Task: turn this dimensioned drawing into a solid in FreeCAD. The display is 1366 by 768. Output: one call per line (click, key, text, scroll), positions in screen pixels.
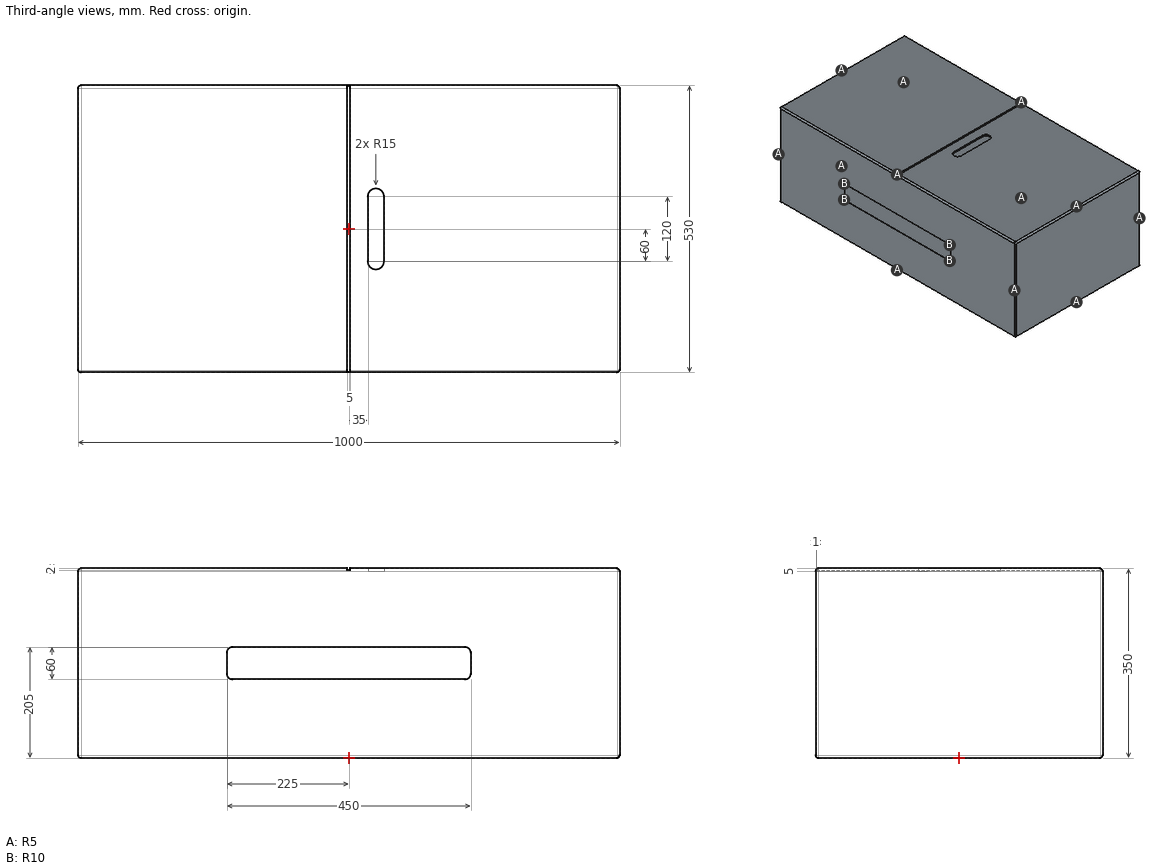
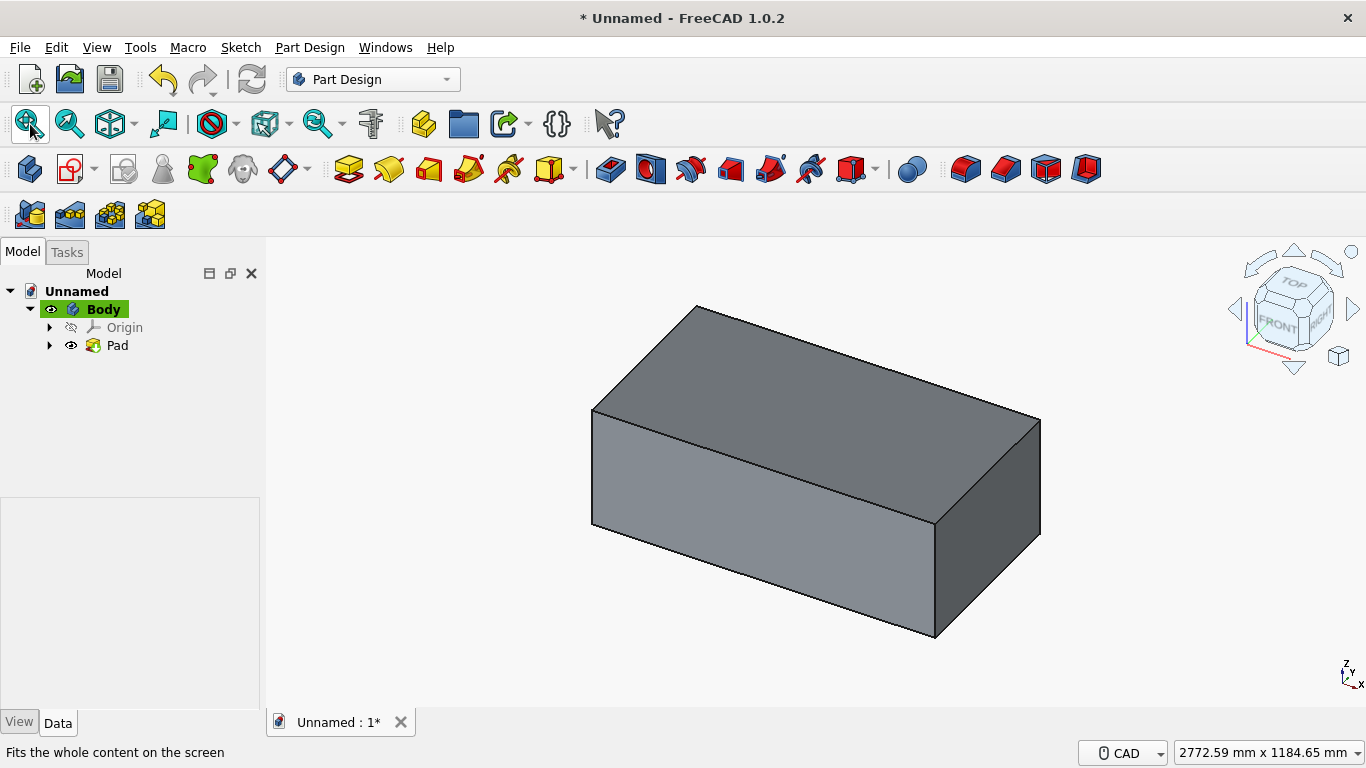
click(865, 430)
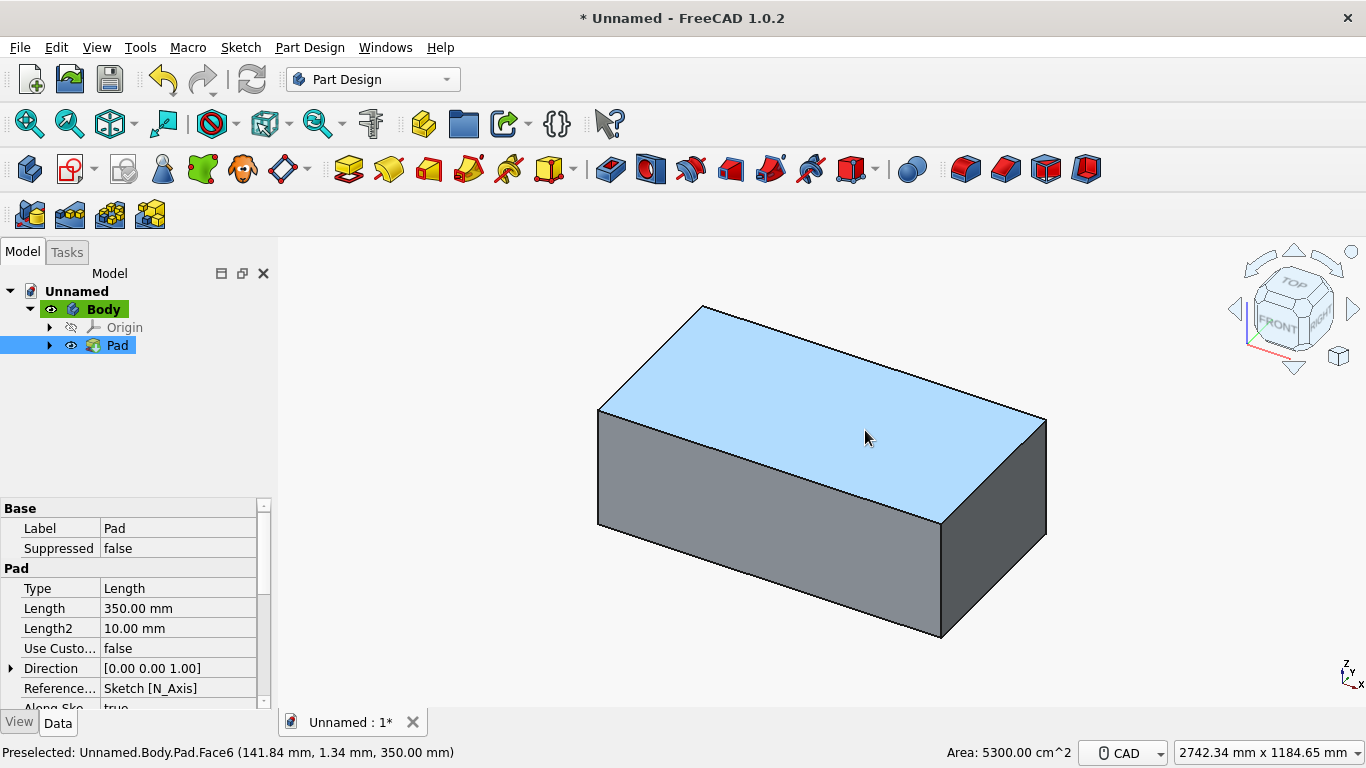
click(941, 580, ctrl)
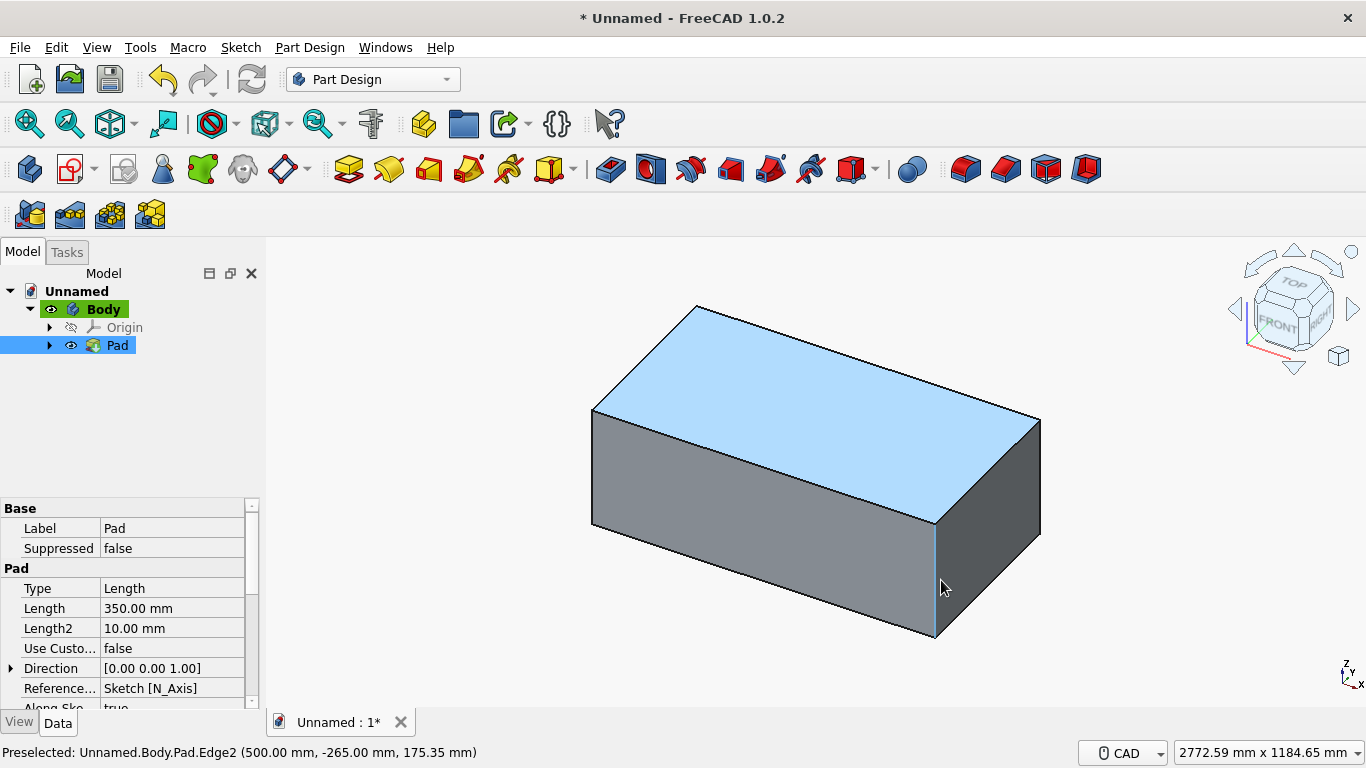
key(0)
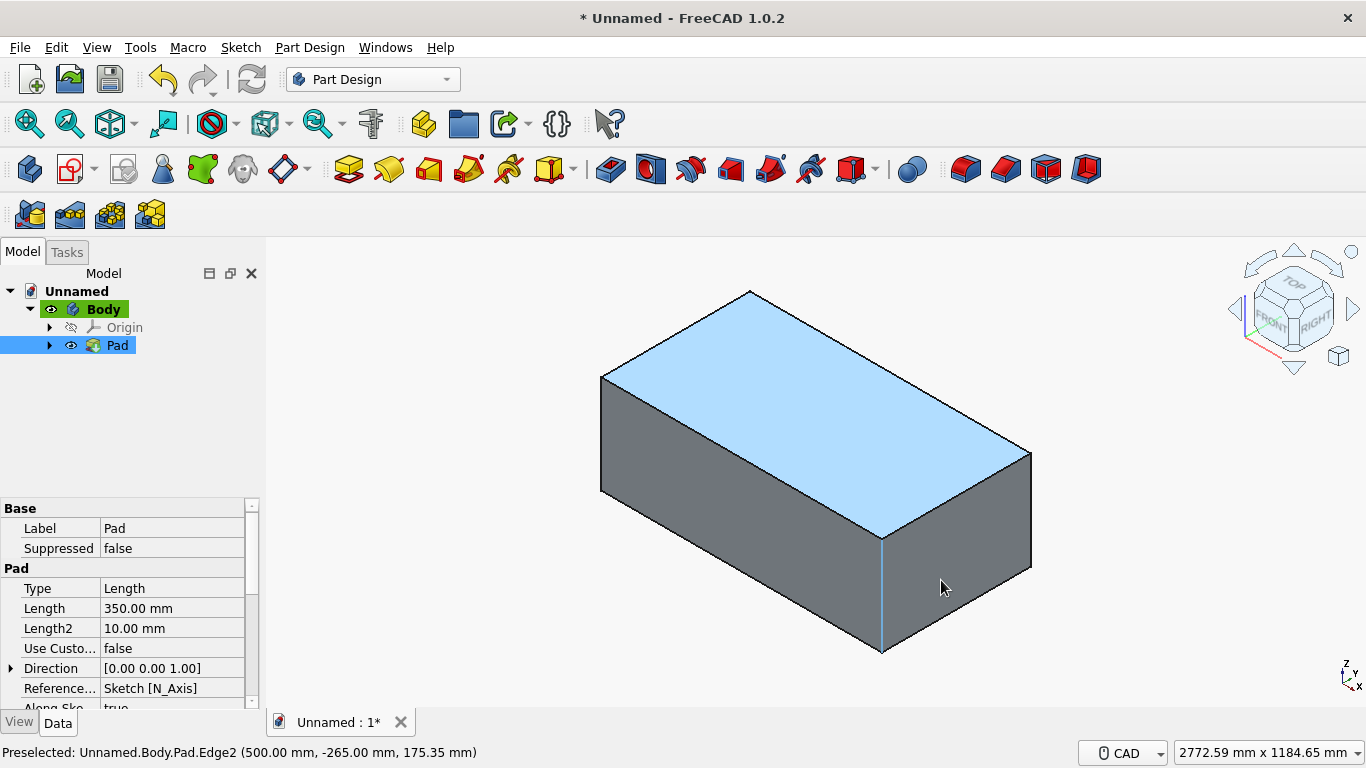
key(2)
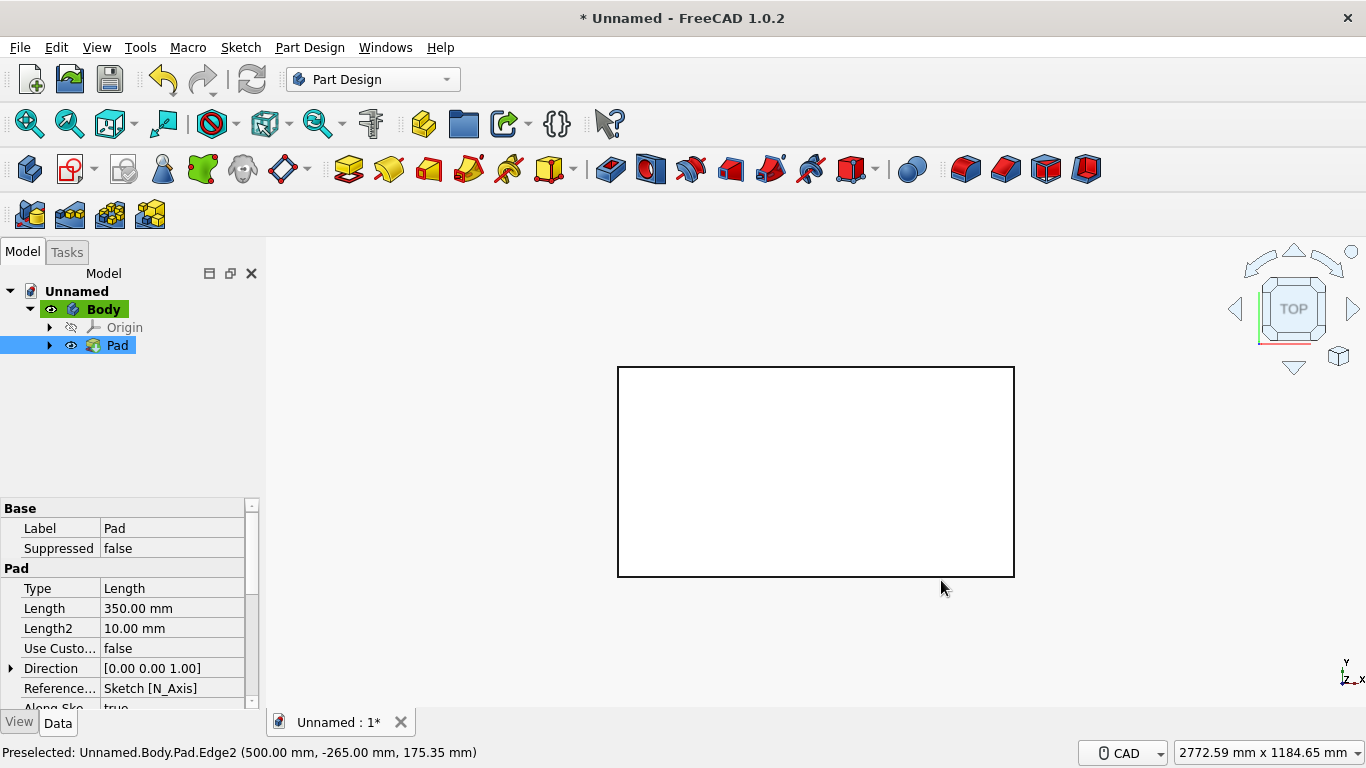
click(30, 124)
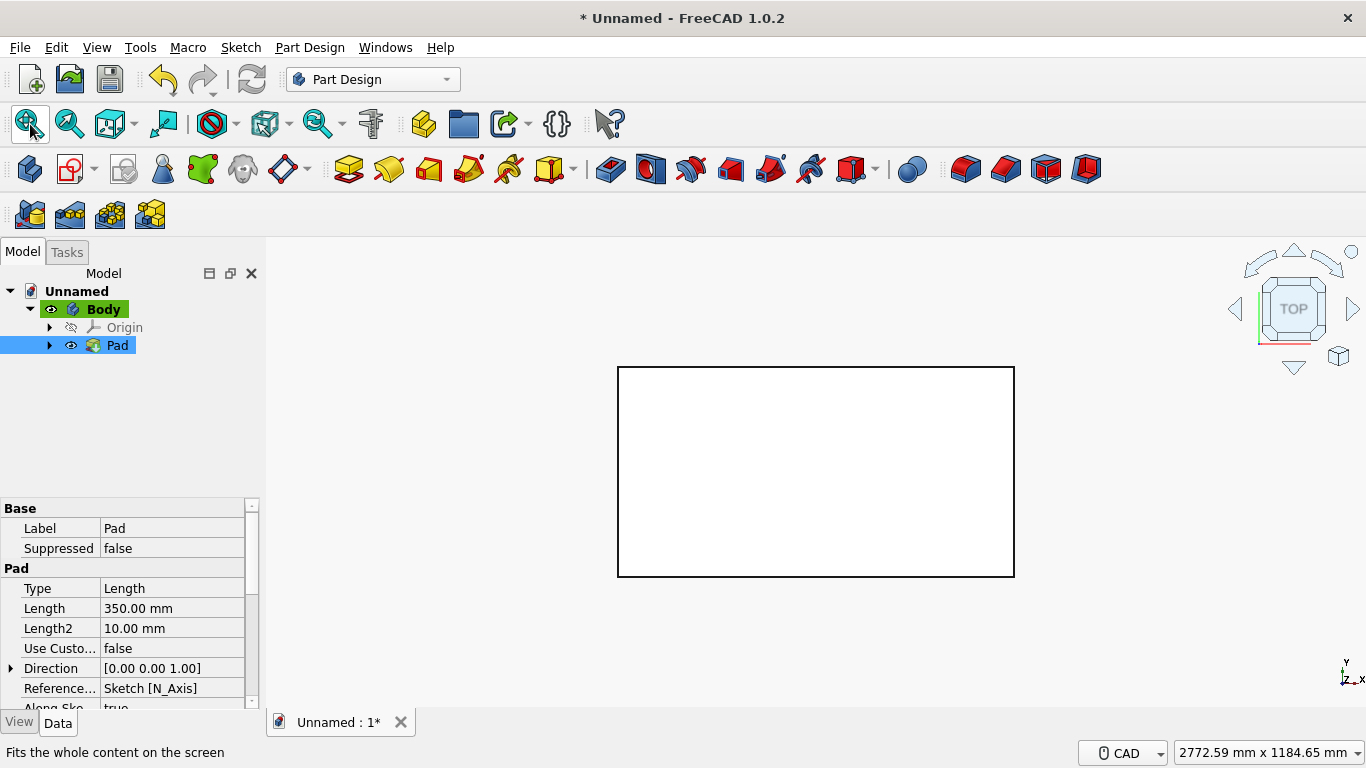
key(1)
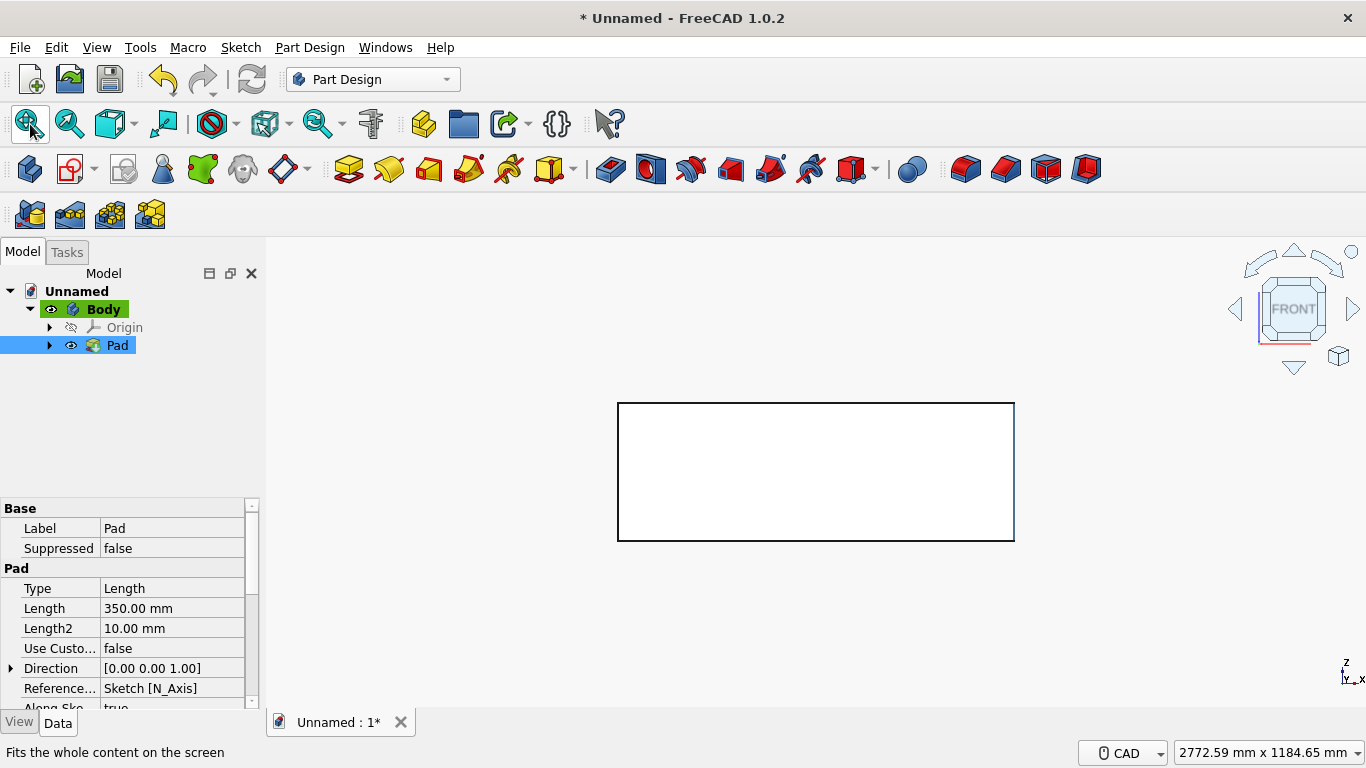
click(30, 124)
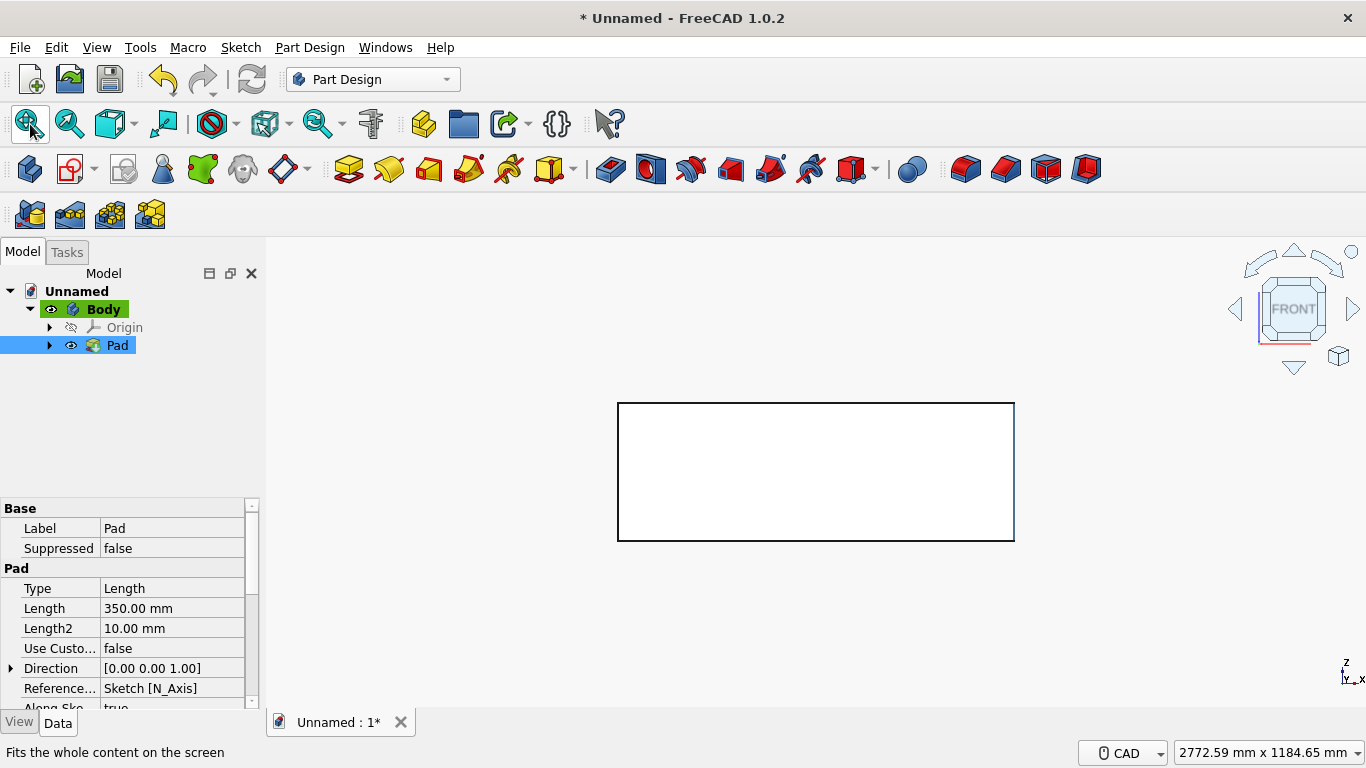
click(618, 471, ctrl)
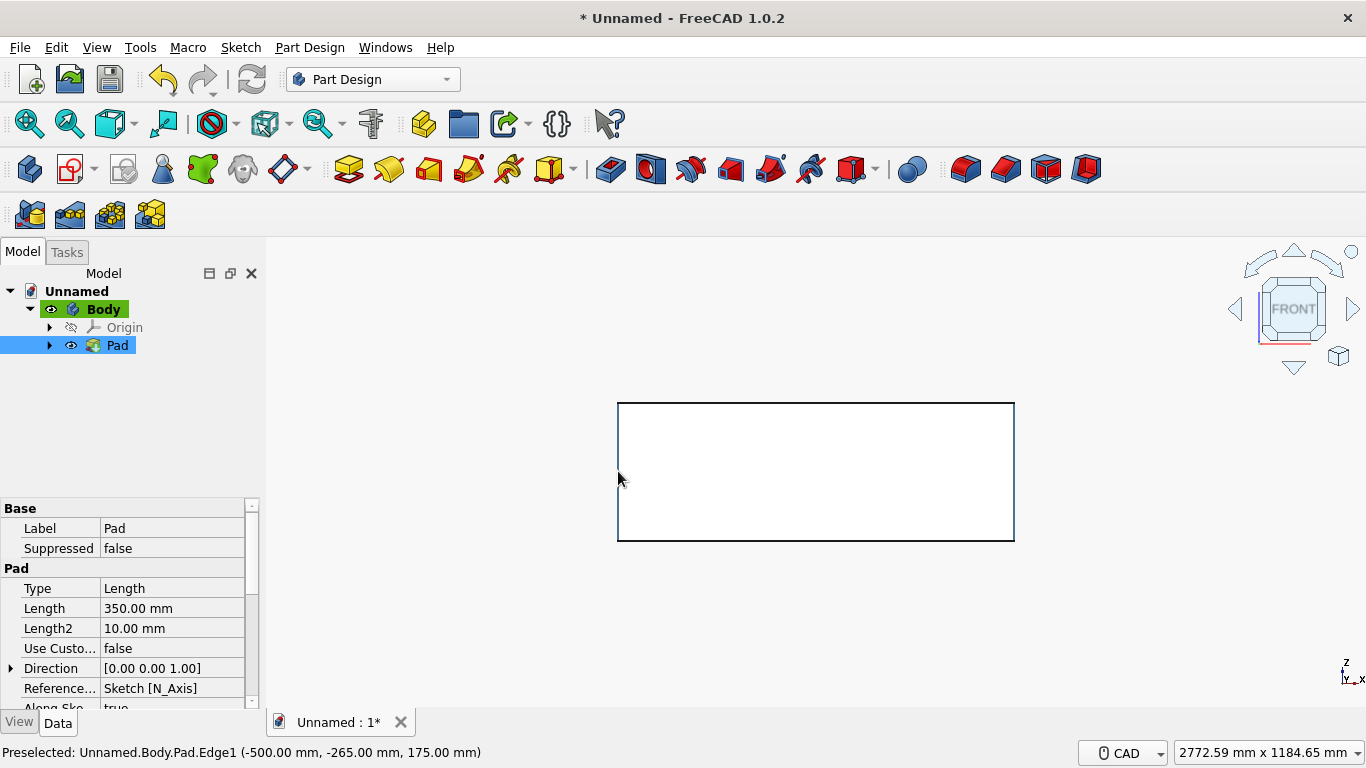
key(3)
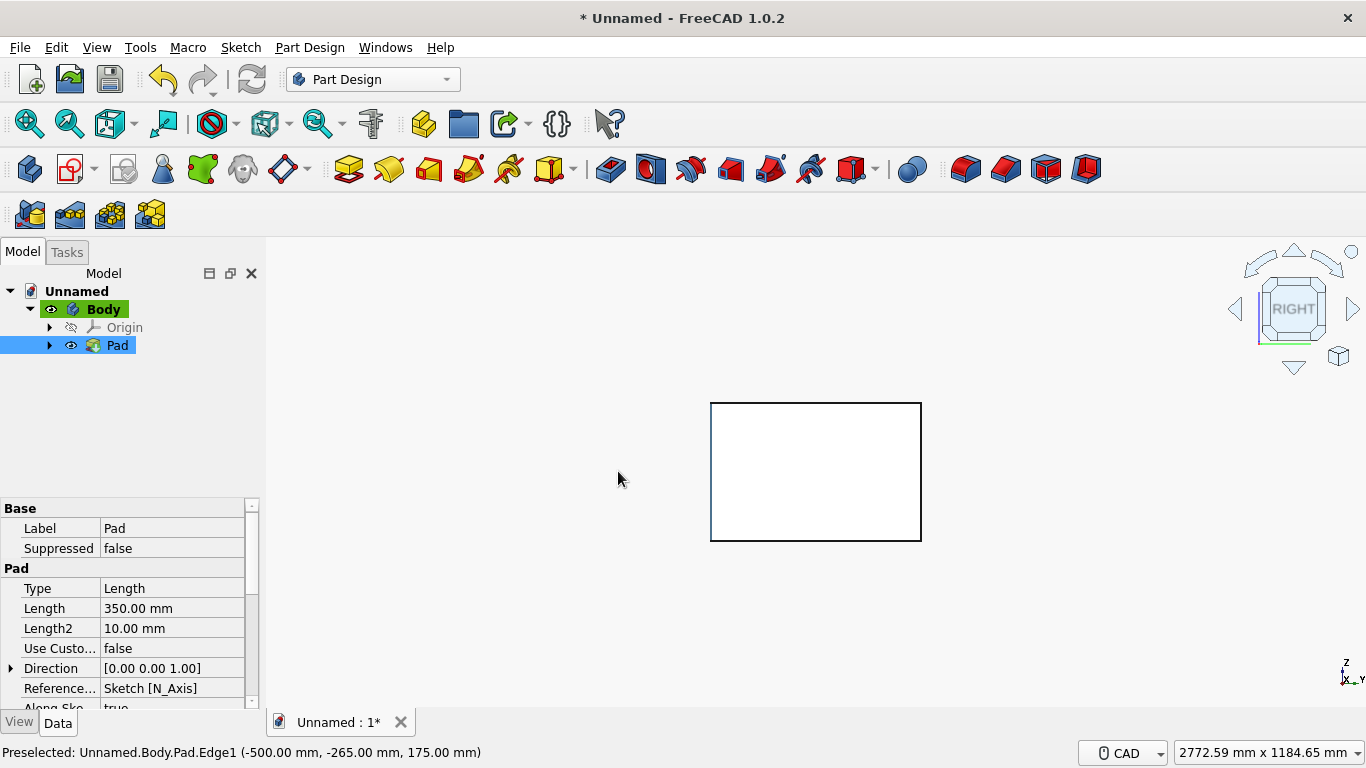
click(30, 124)